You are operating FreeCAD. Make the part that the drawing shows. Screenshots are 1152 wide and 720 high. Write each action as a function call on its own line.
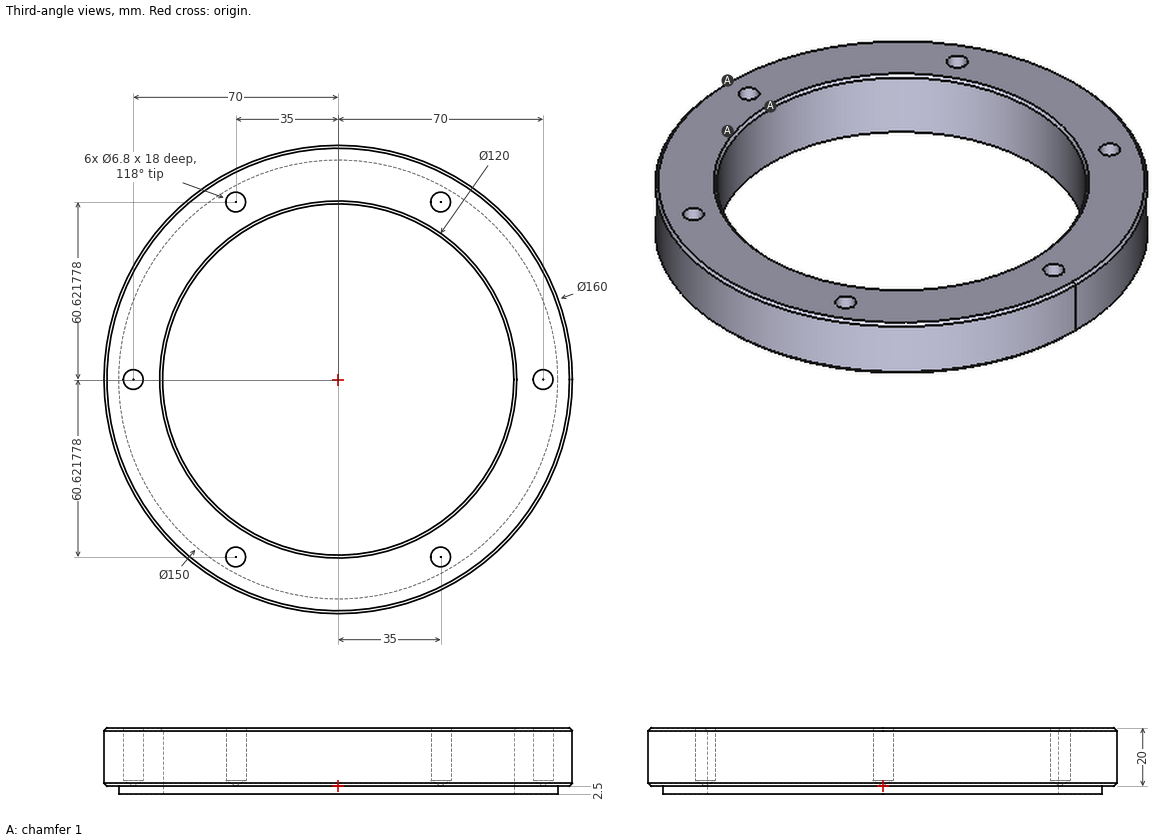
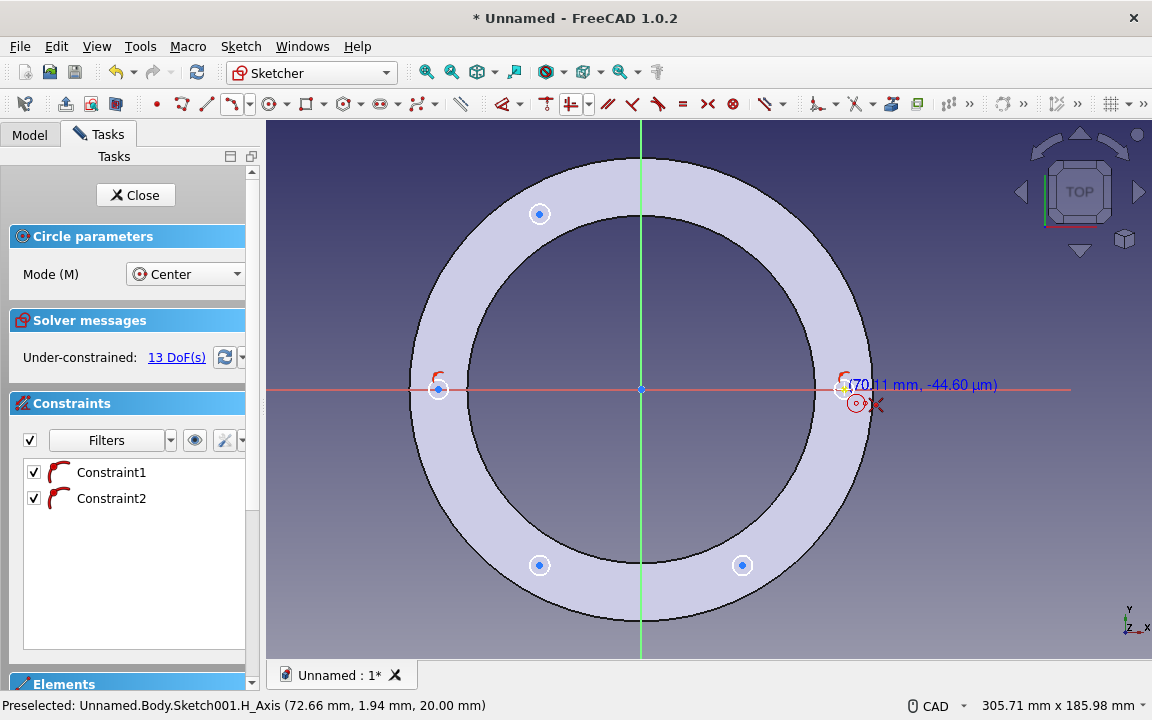
scroll(743, 214, up, 5)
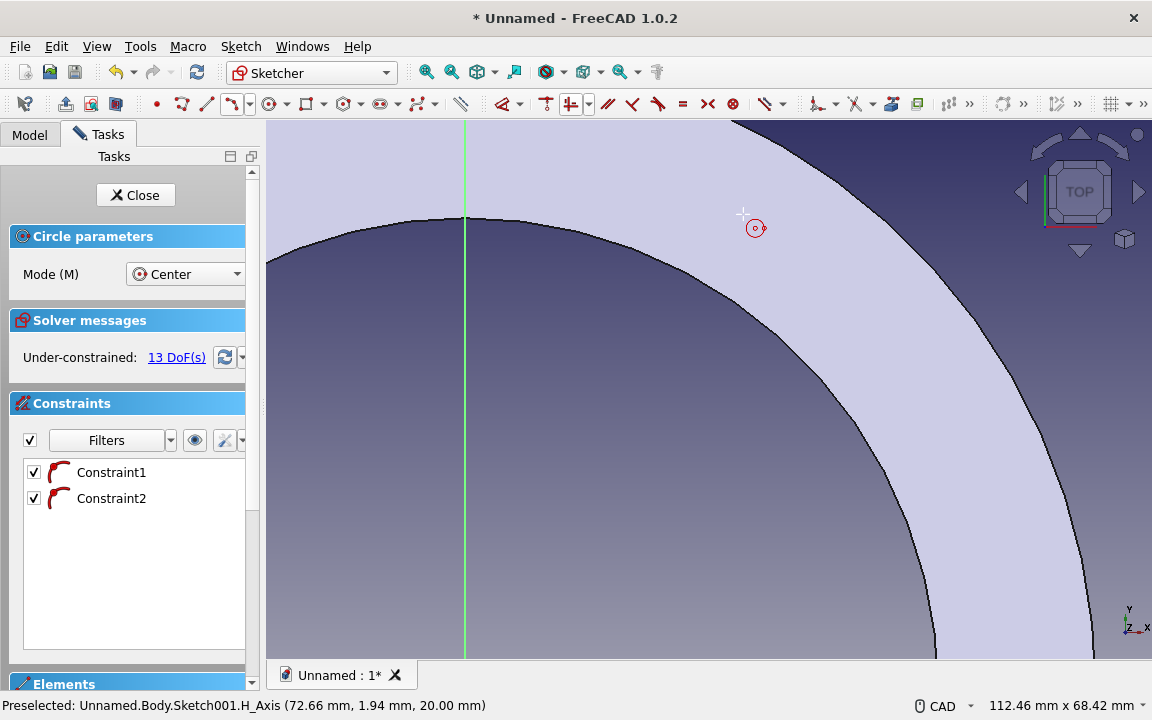
click(741, 213)
click(760, 194)
key(Escape)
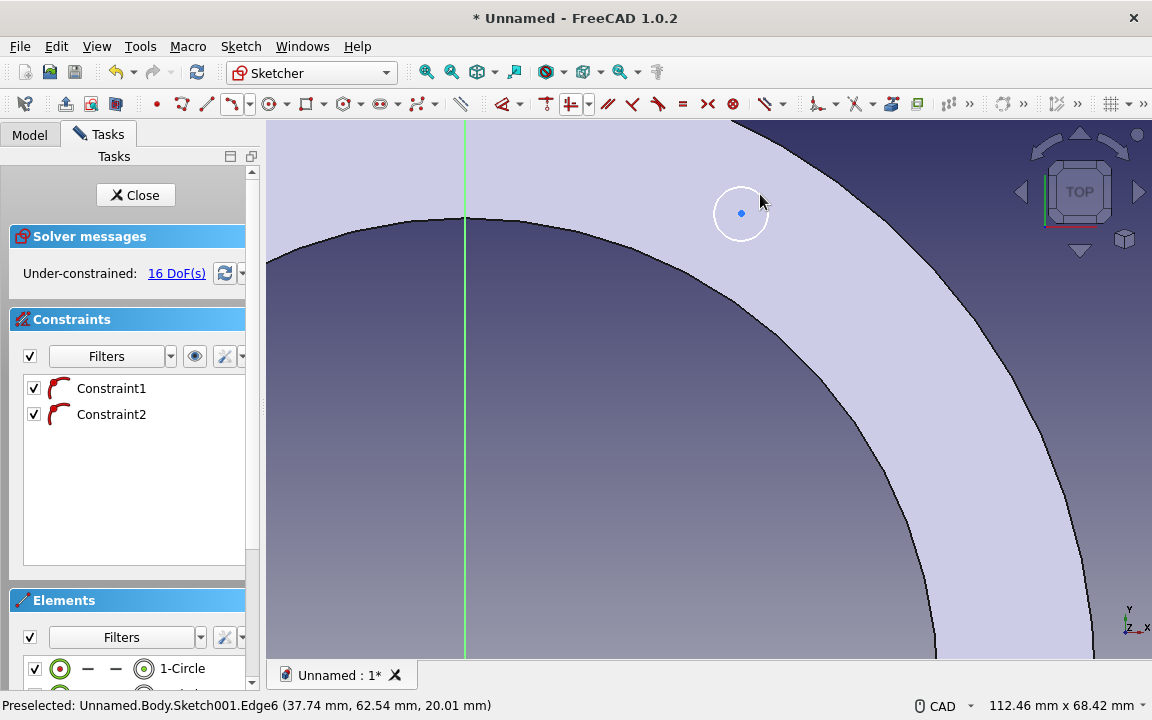
scroll(742, 214, down, 5)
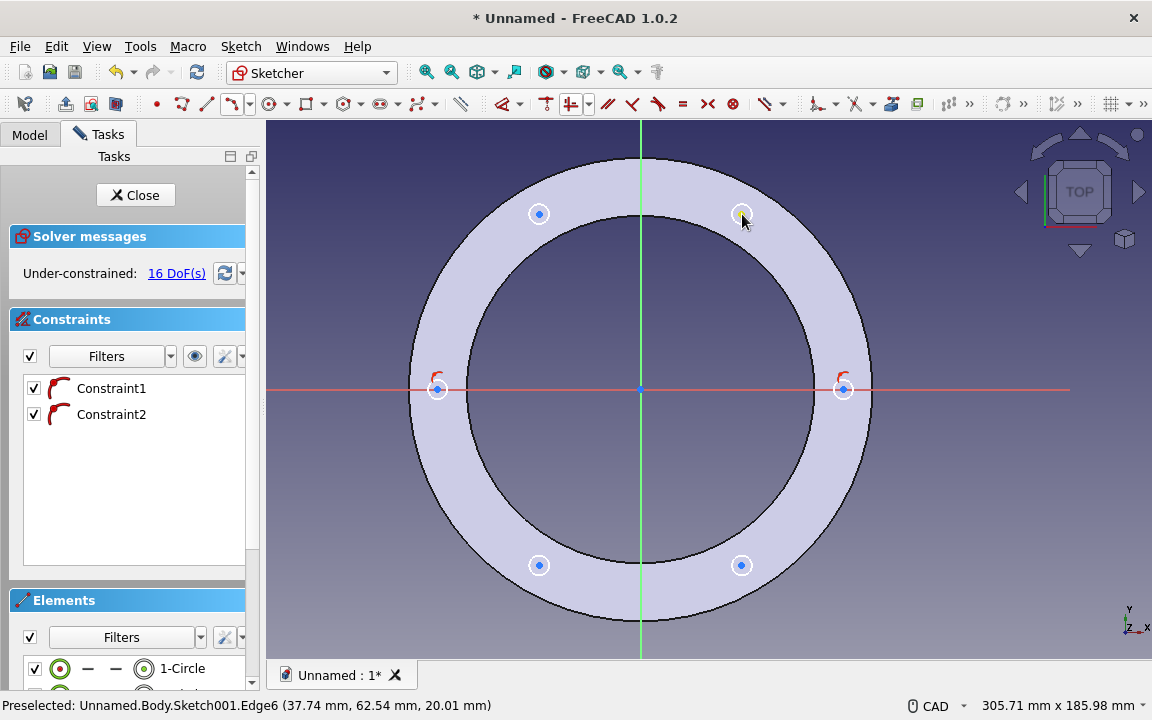
scroll(546, 207, up, 2)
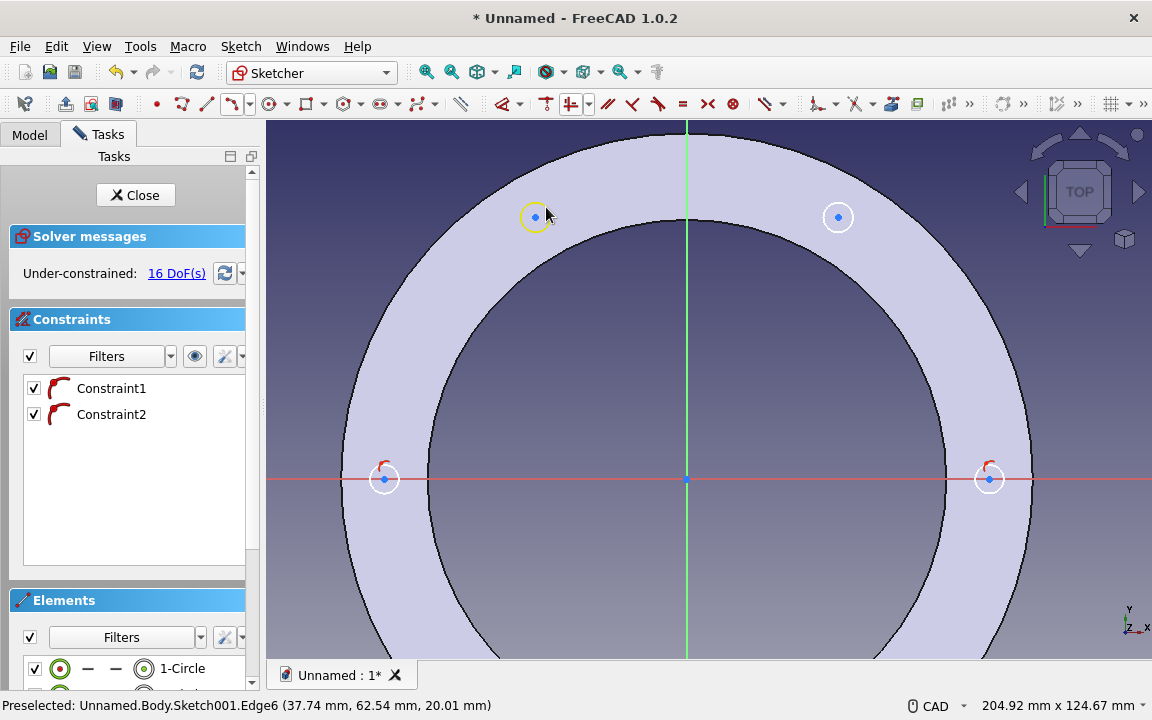
click(546, 207)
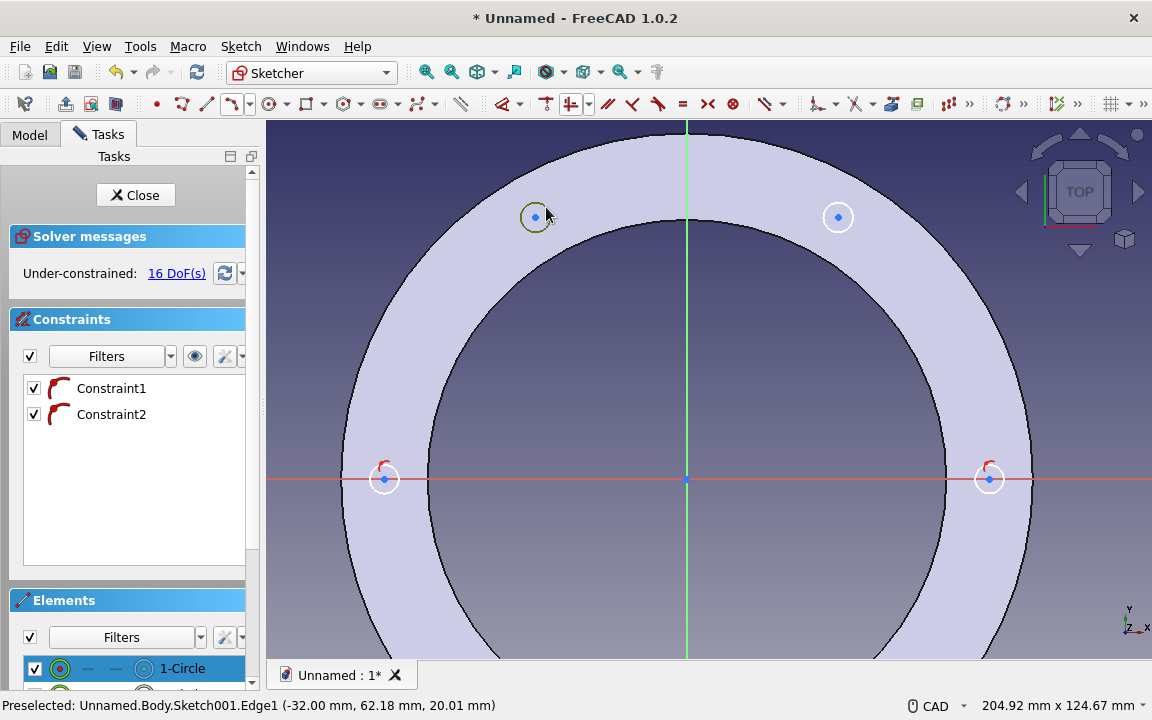
scroll(394, 469, up, 2)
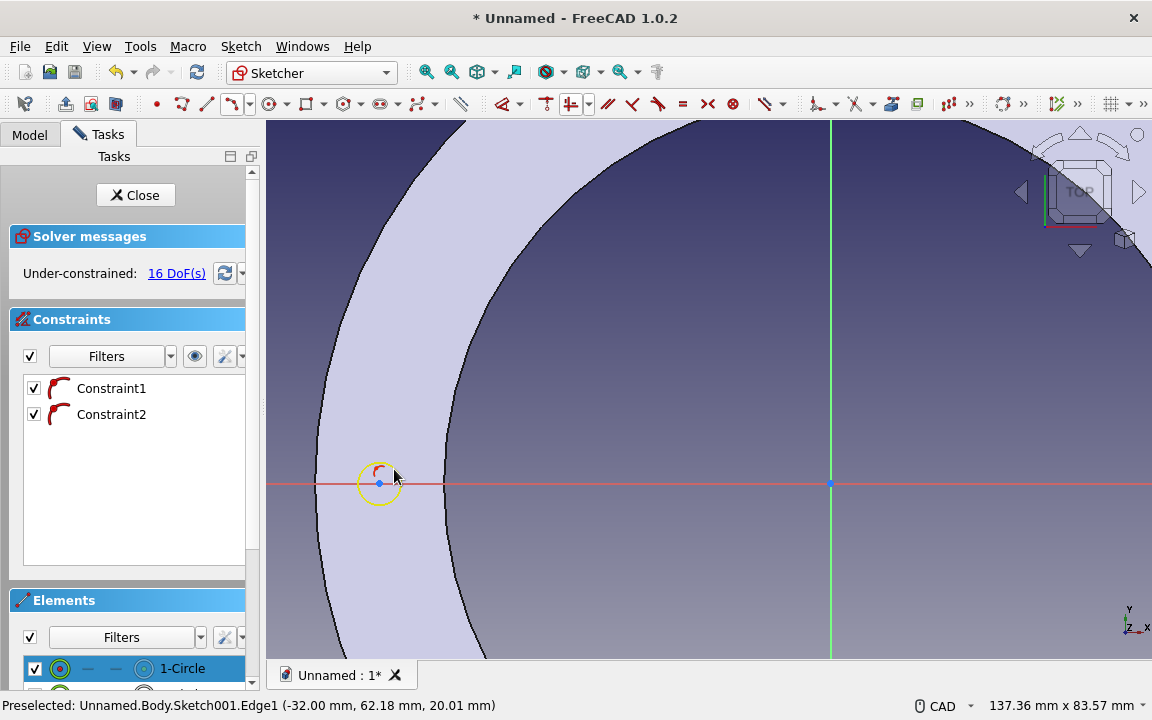
click(395, 469)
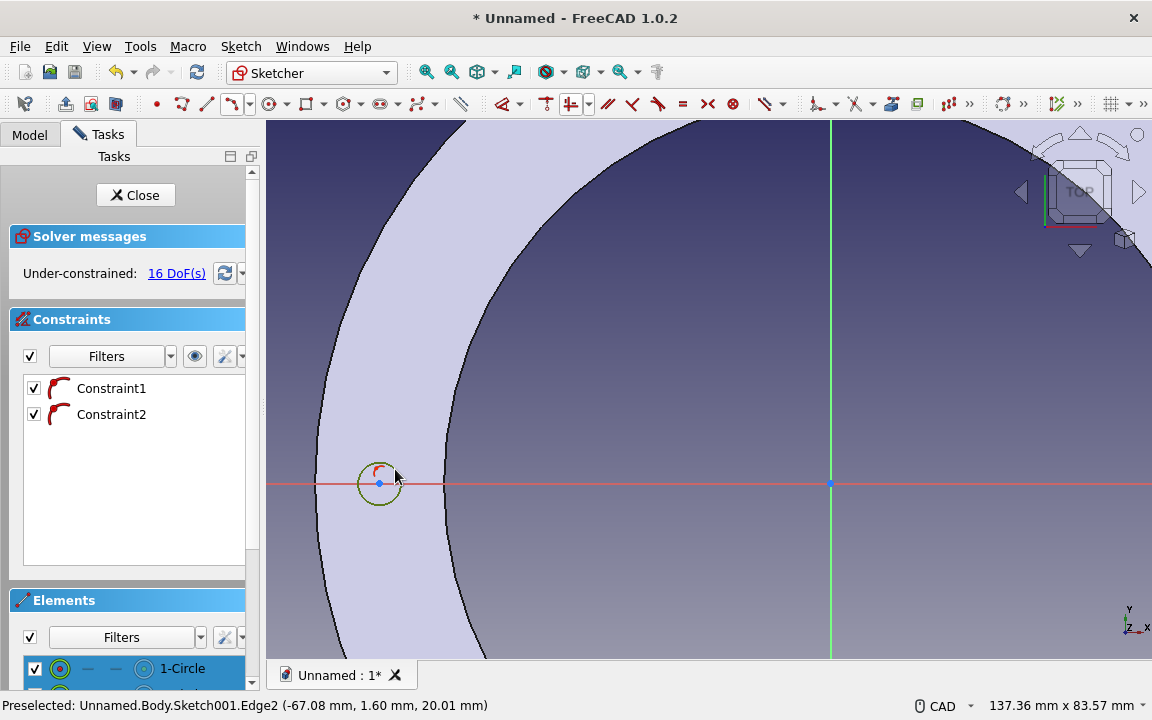
scroll(485, 312, down, 4)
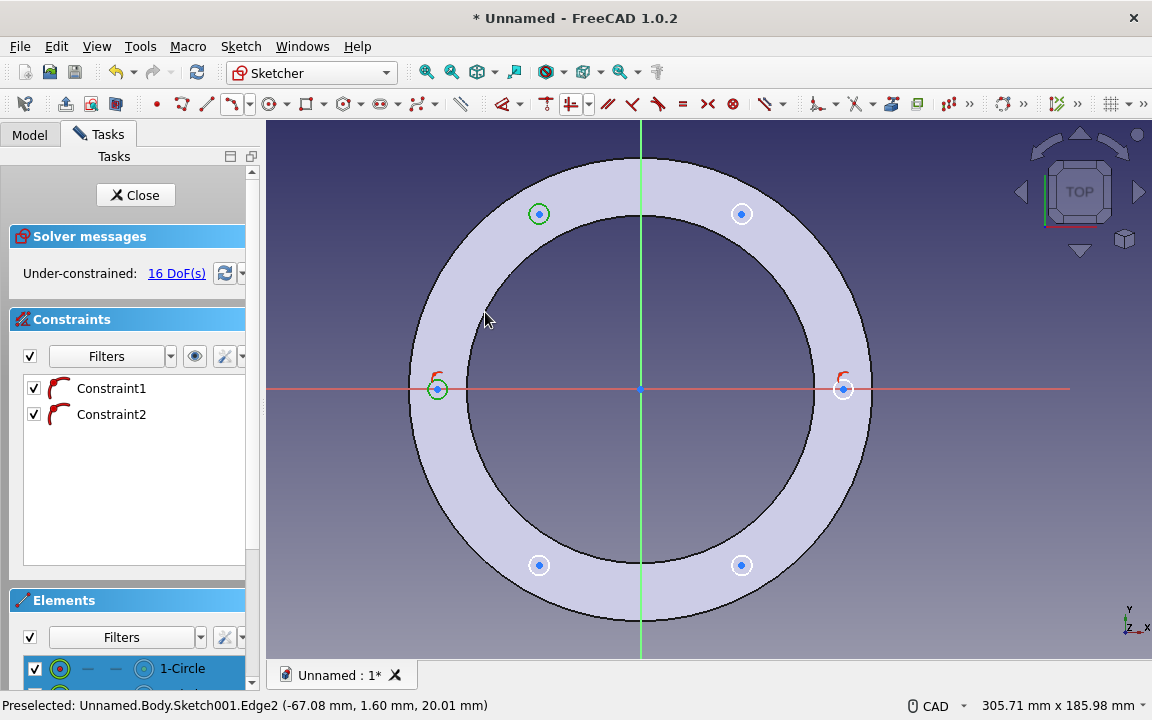
scroll(546, 558, up, 2)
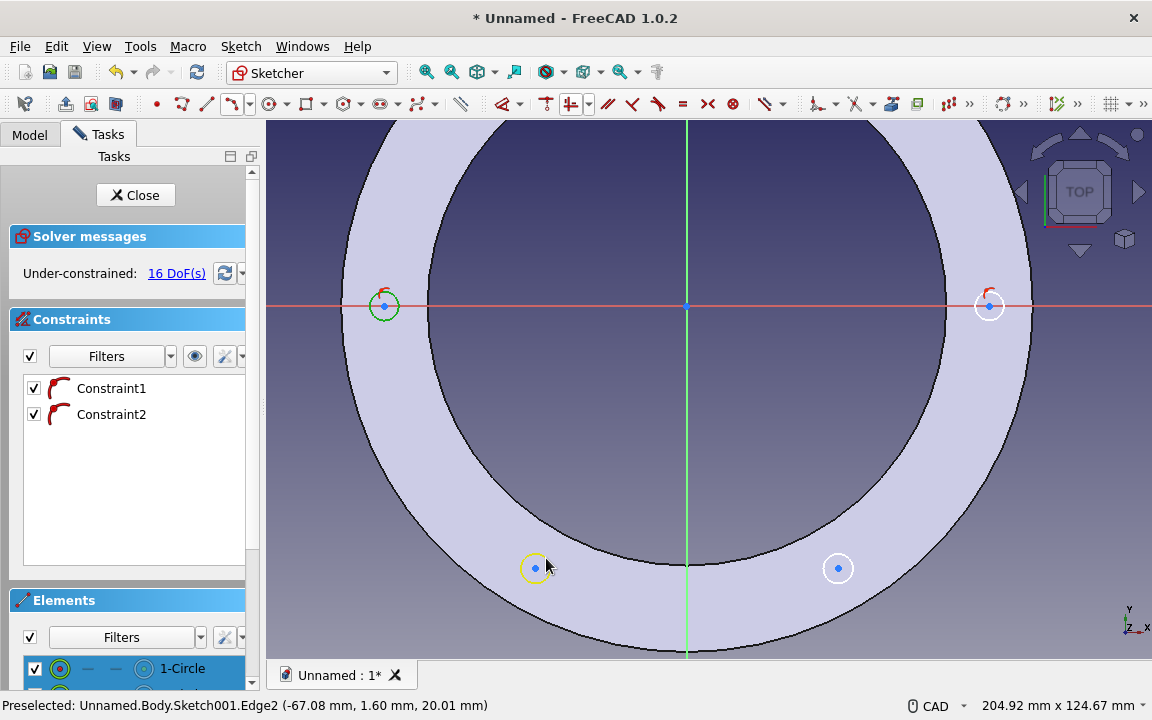
click(546, 558)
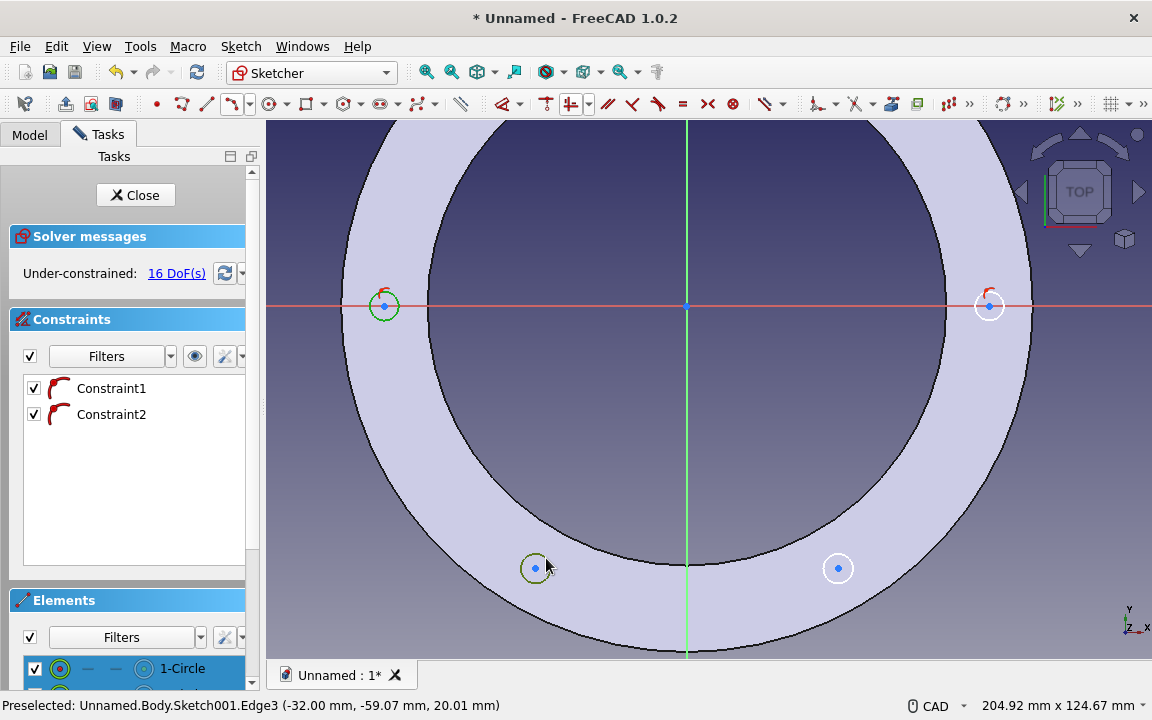
click(849, 558)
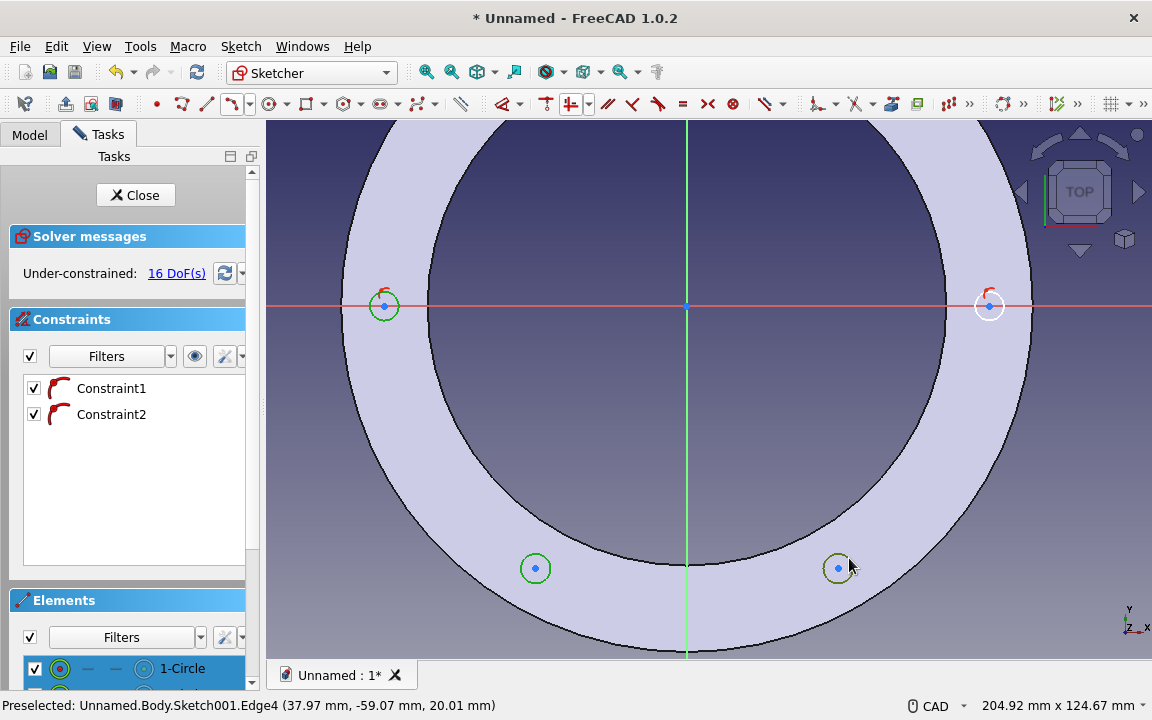
scroll(979, 296, up, 2)